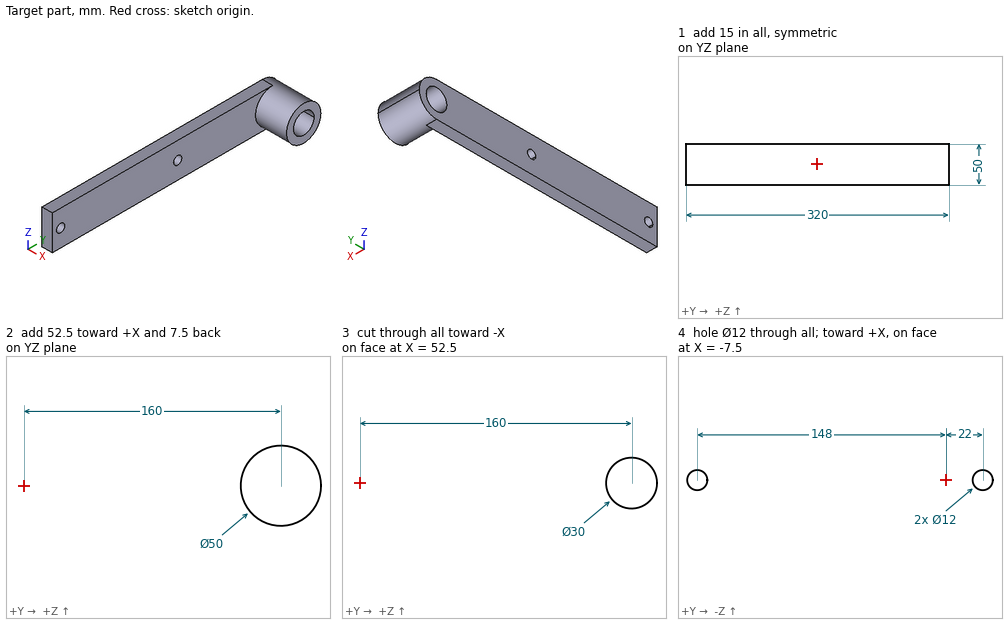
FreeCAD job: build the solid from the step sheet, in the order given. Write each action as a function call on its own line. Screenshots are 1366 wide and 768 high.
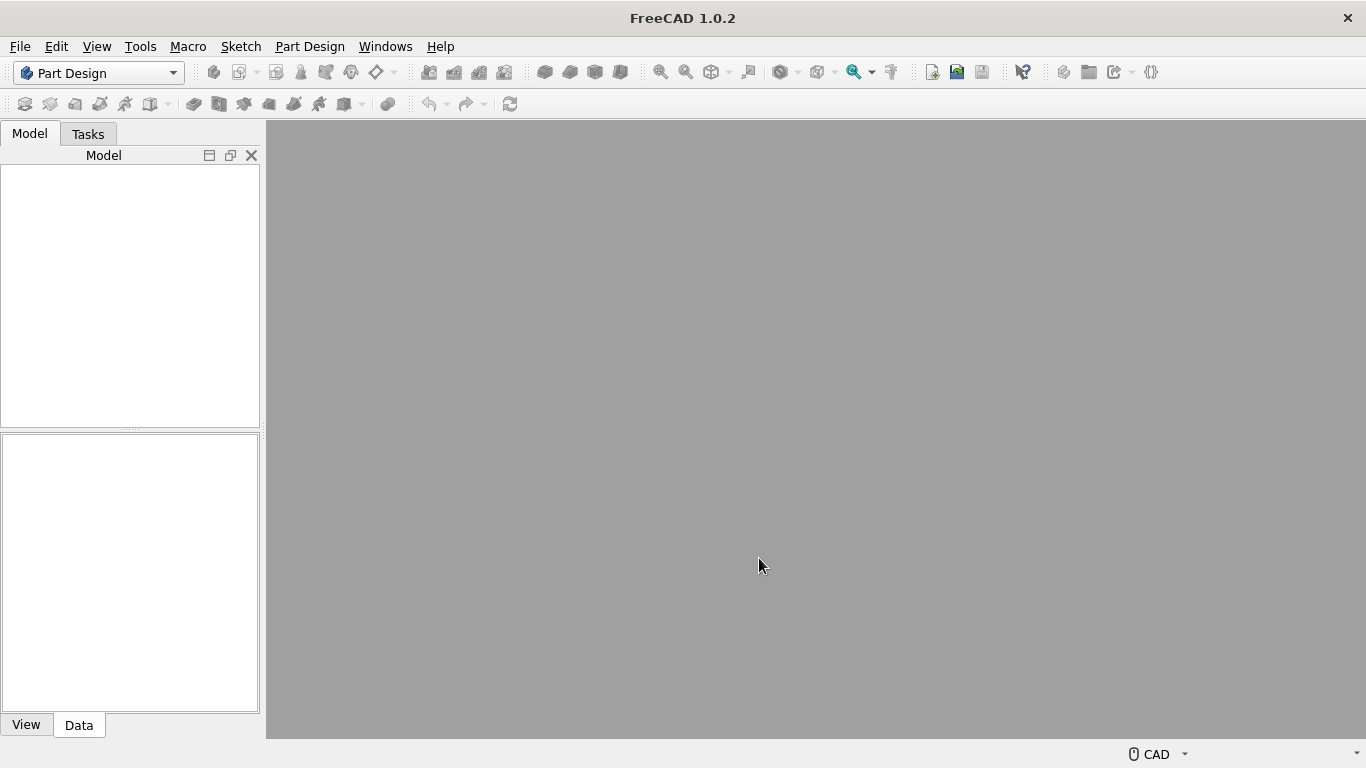
click(932, 72)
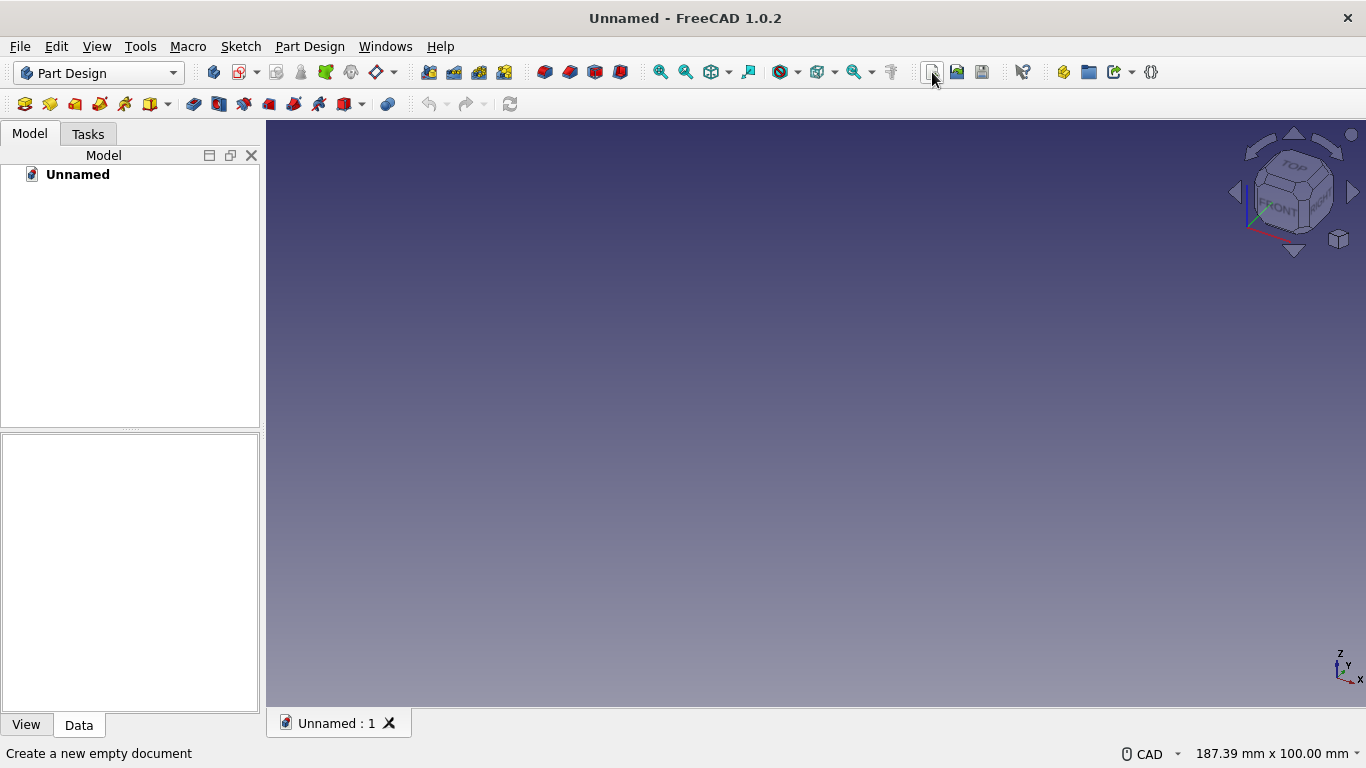
click(238, 72)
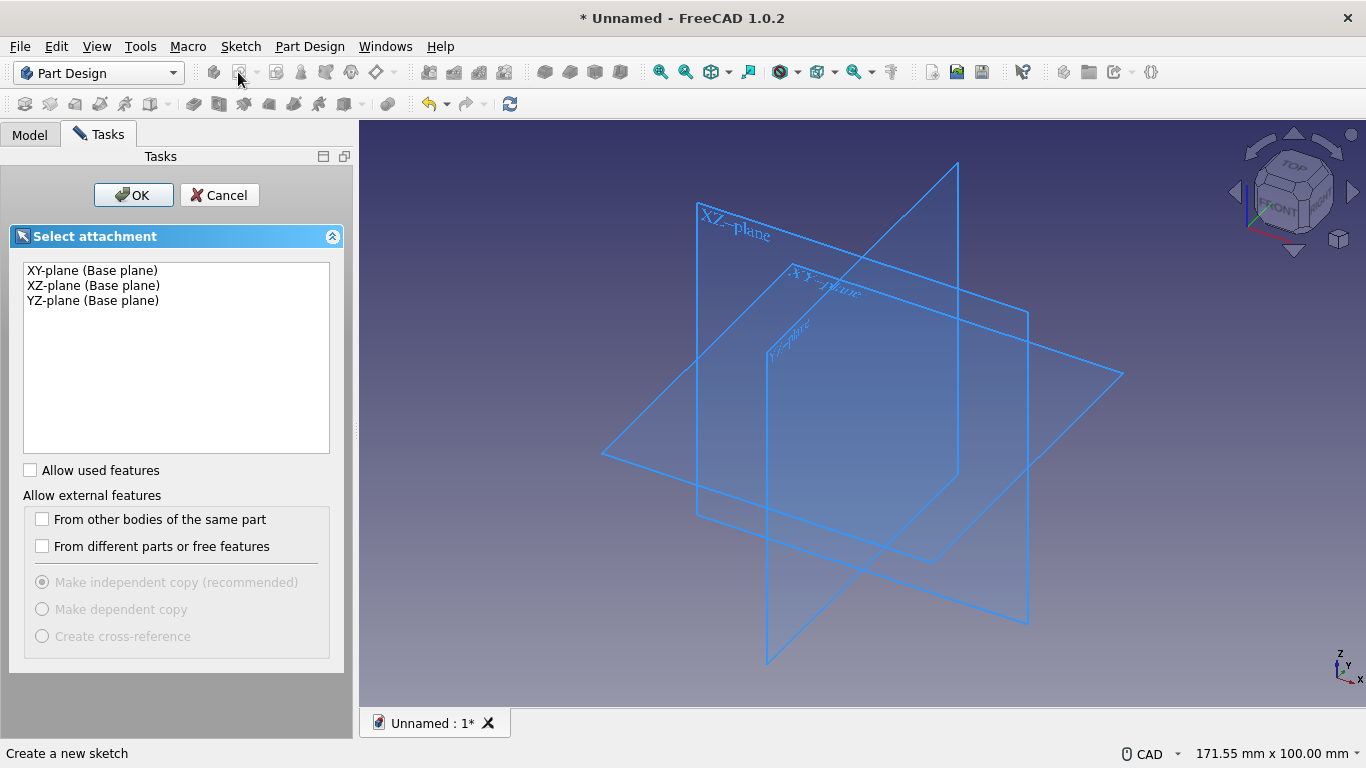
click(84, 300)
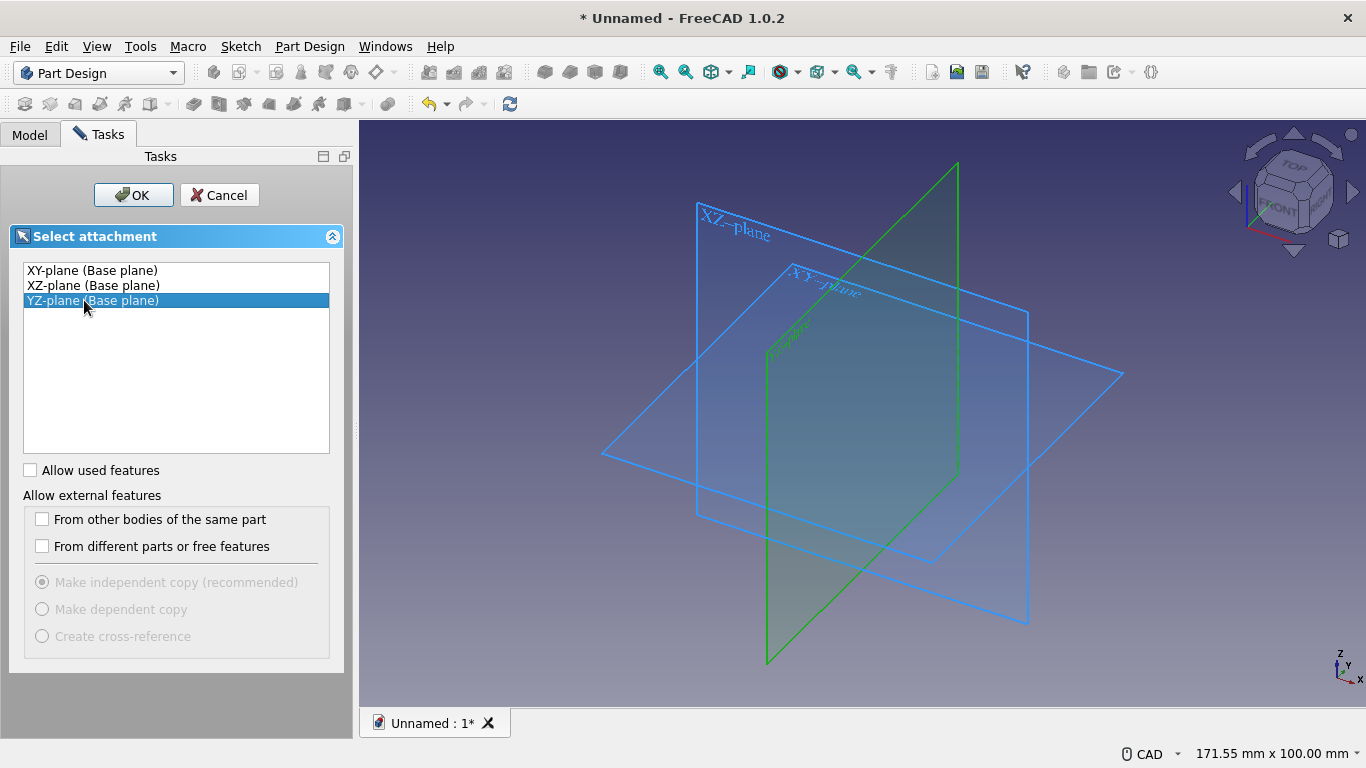
click(134, 195)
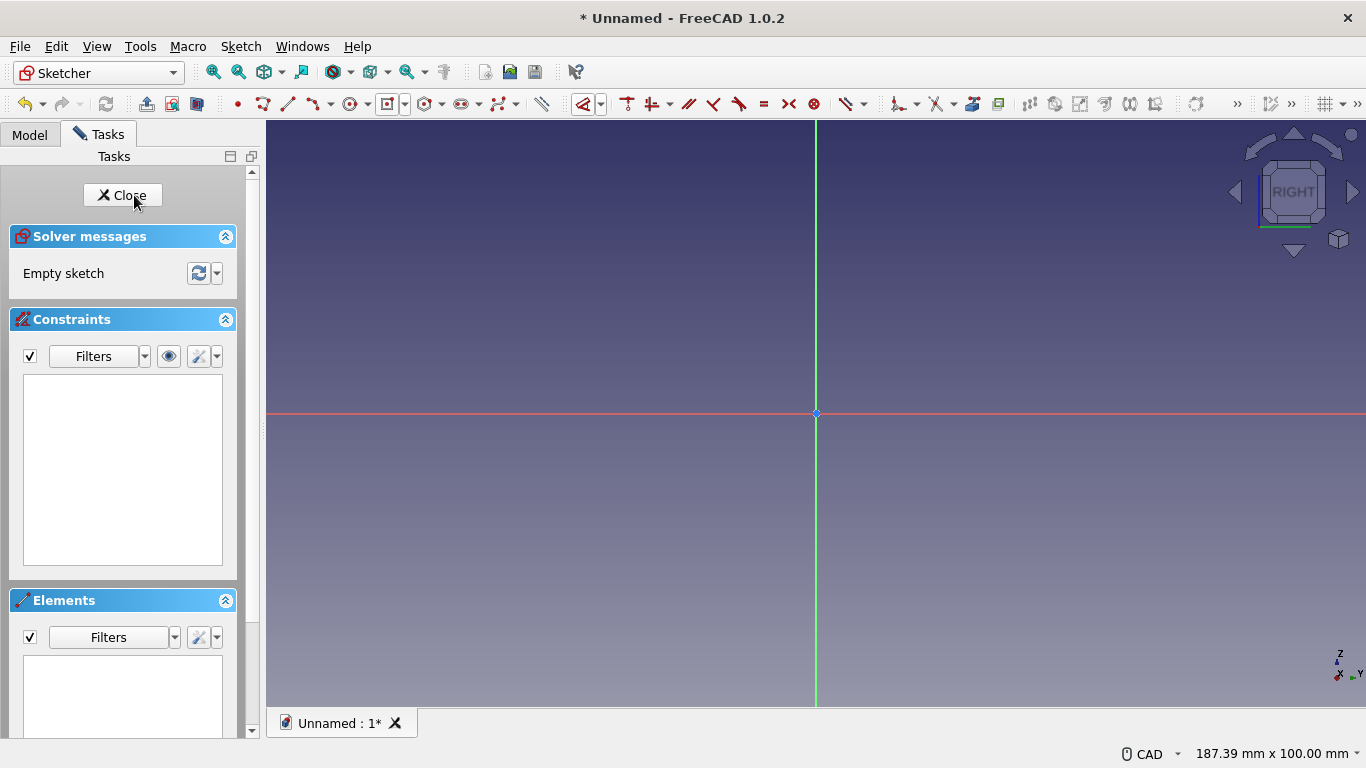
scroll(708, 414, down, 5)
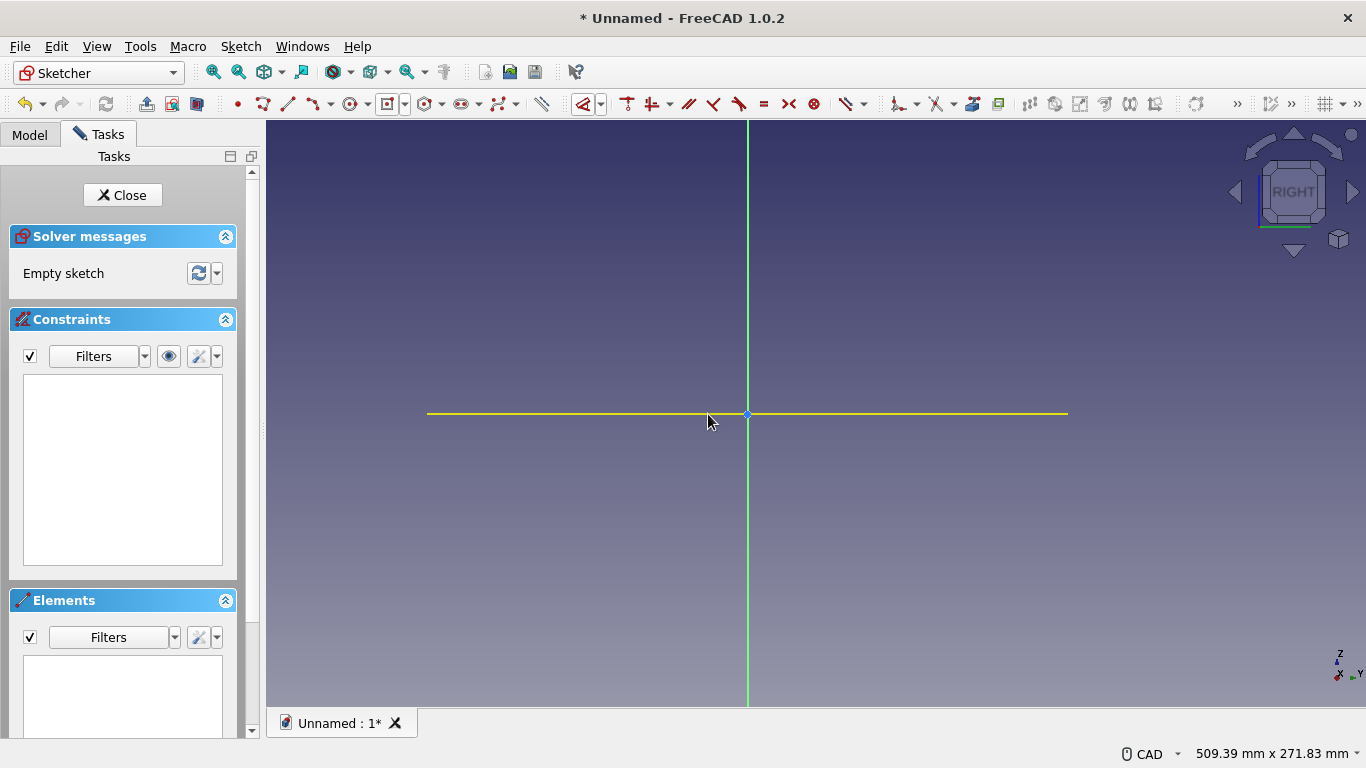
click(386, 104)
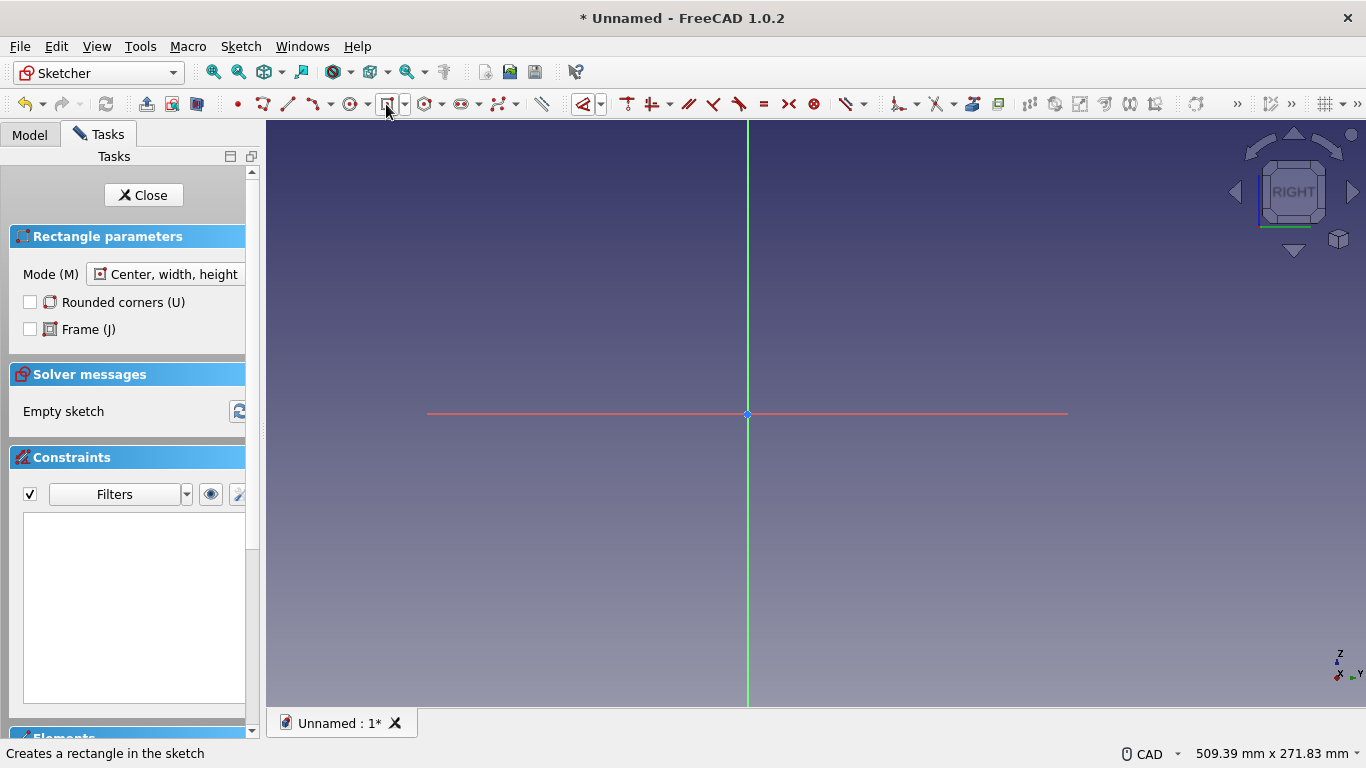
click(748, 414)
click(1093, 360)
key(Escape)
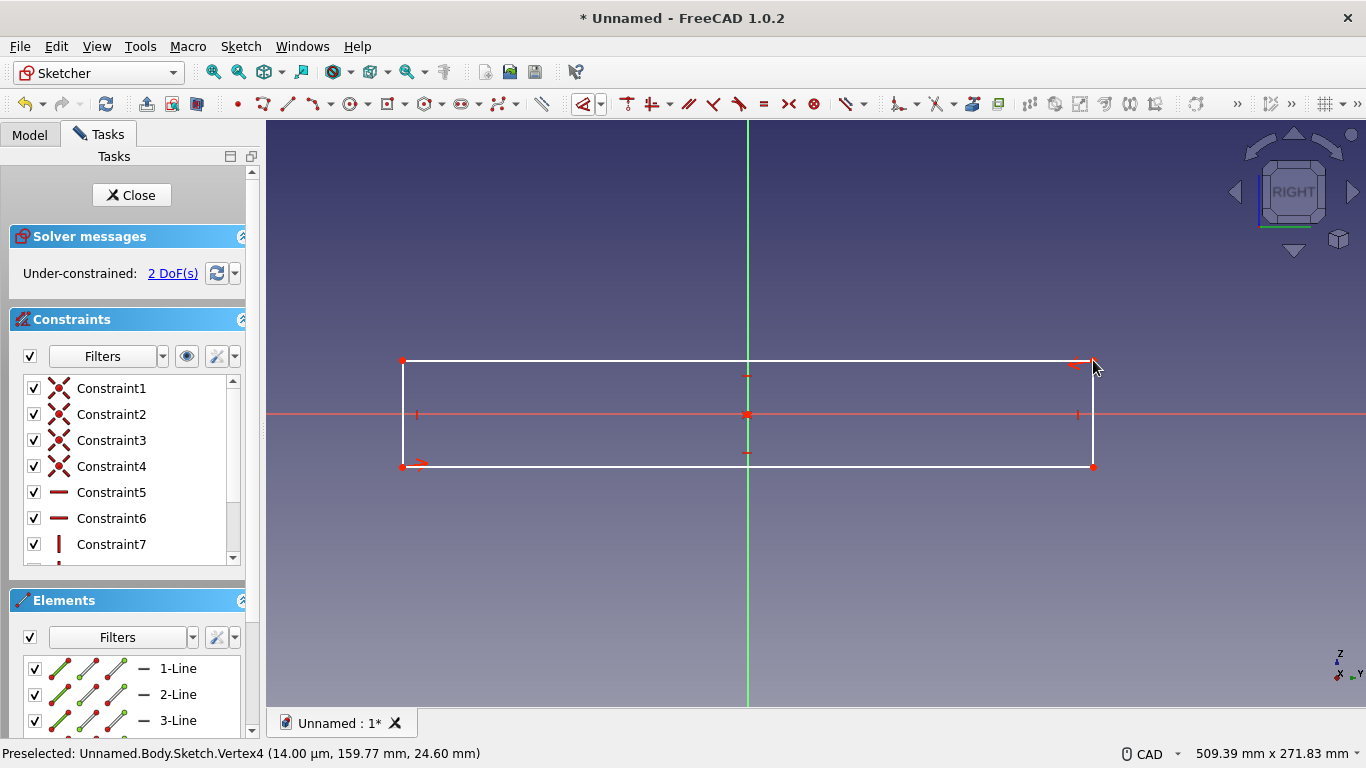
click(582, 104)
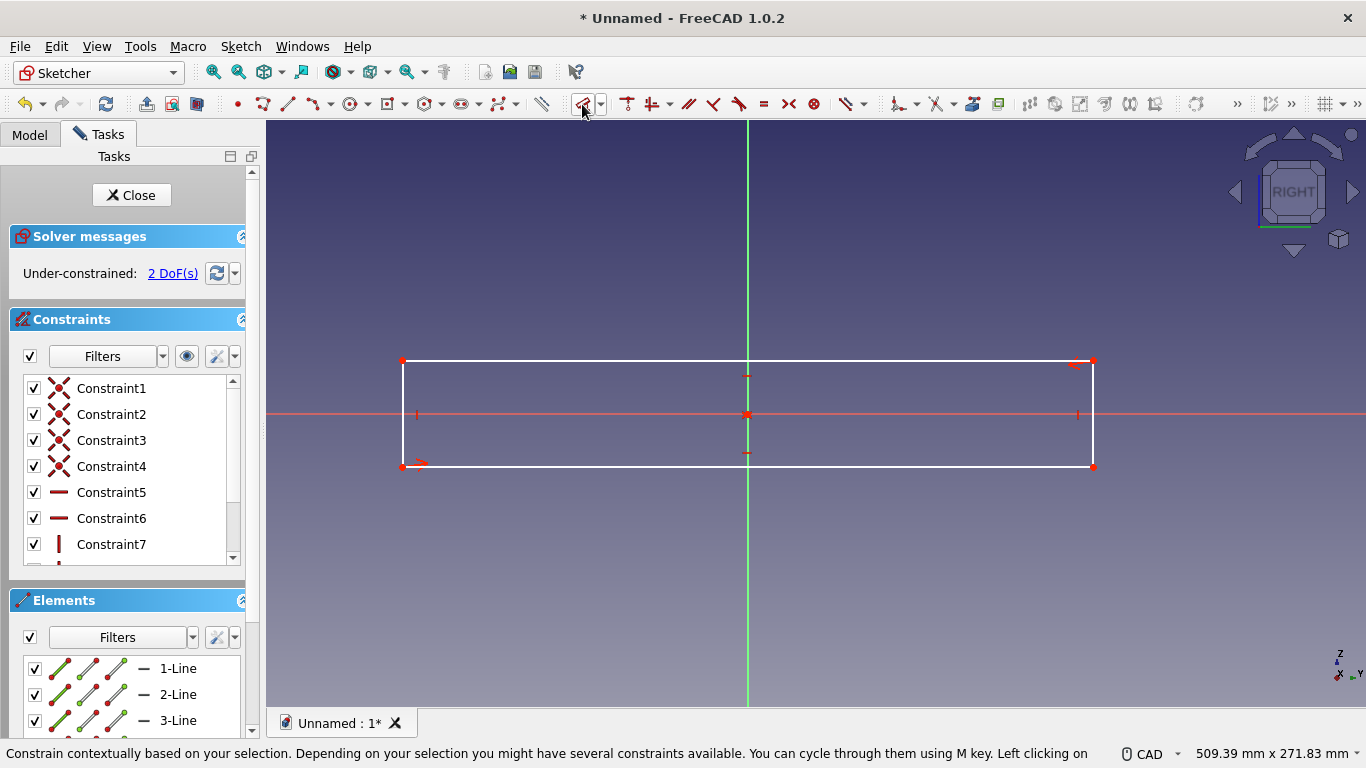
click(1093, 435)
click(1127, 390)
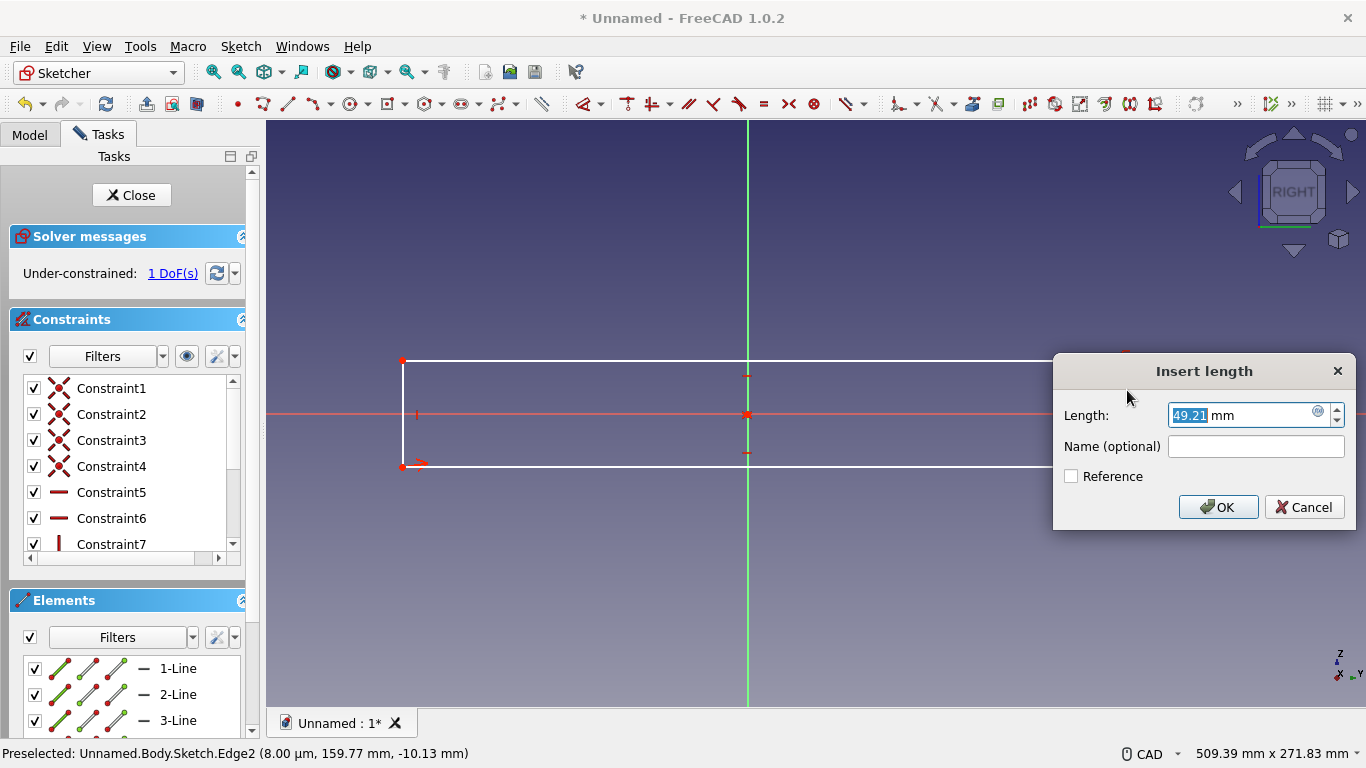
text(50)
key(Return)